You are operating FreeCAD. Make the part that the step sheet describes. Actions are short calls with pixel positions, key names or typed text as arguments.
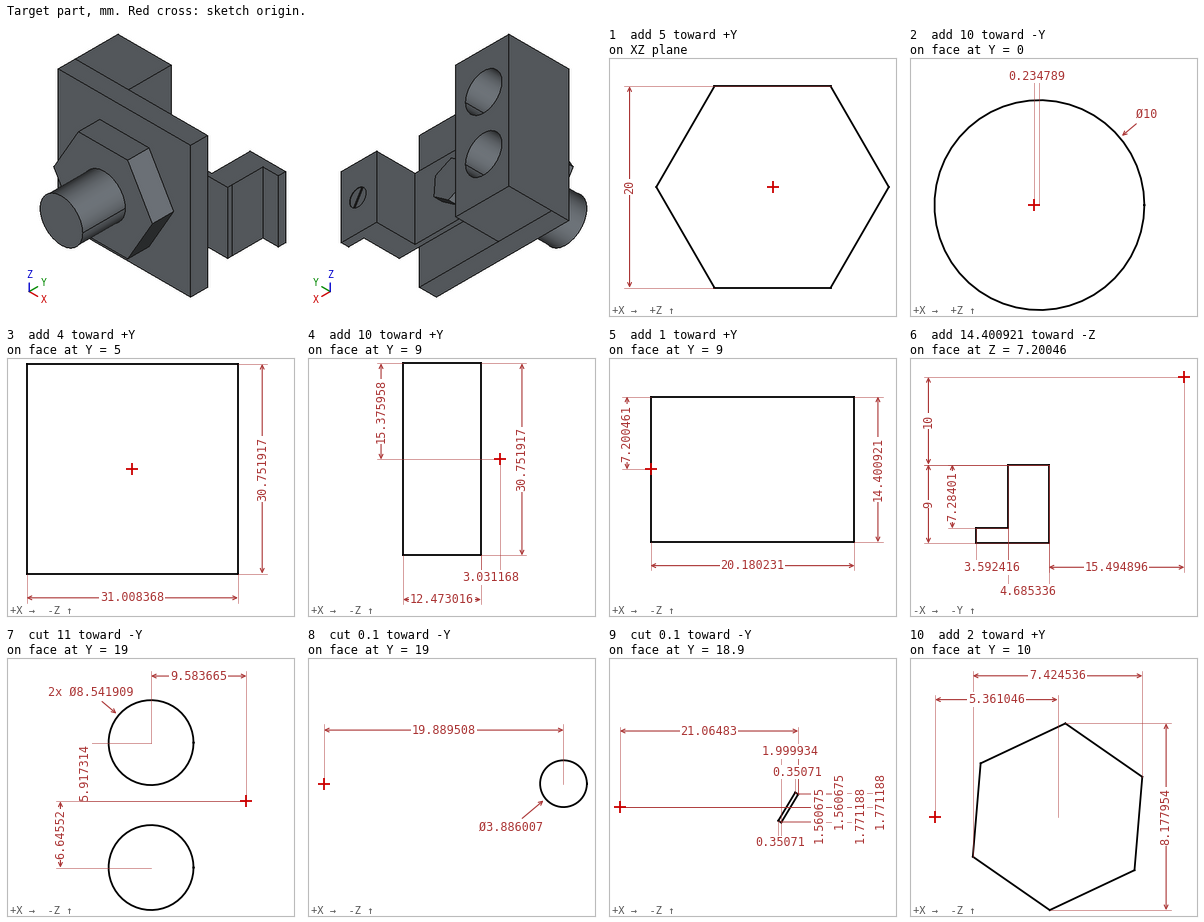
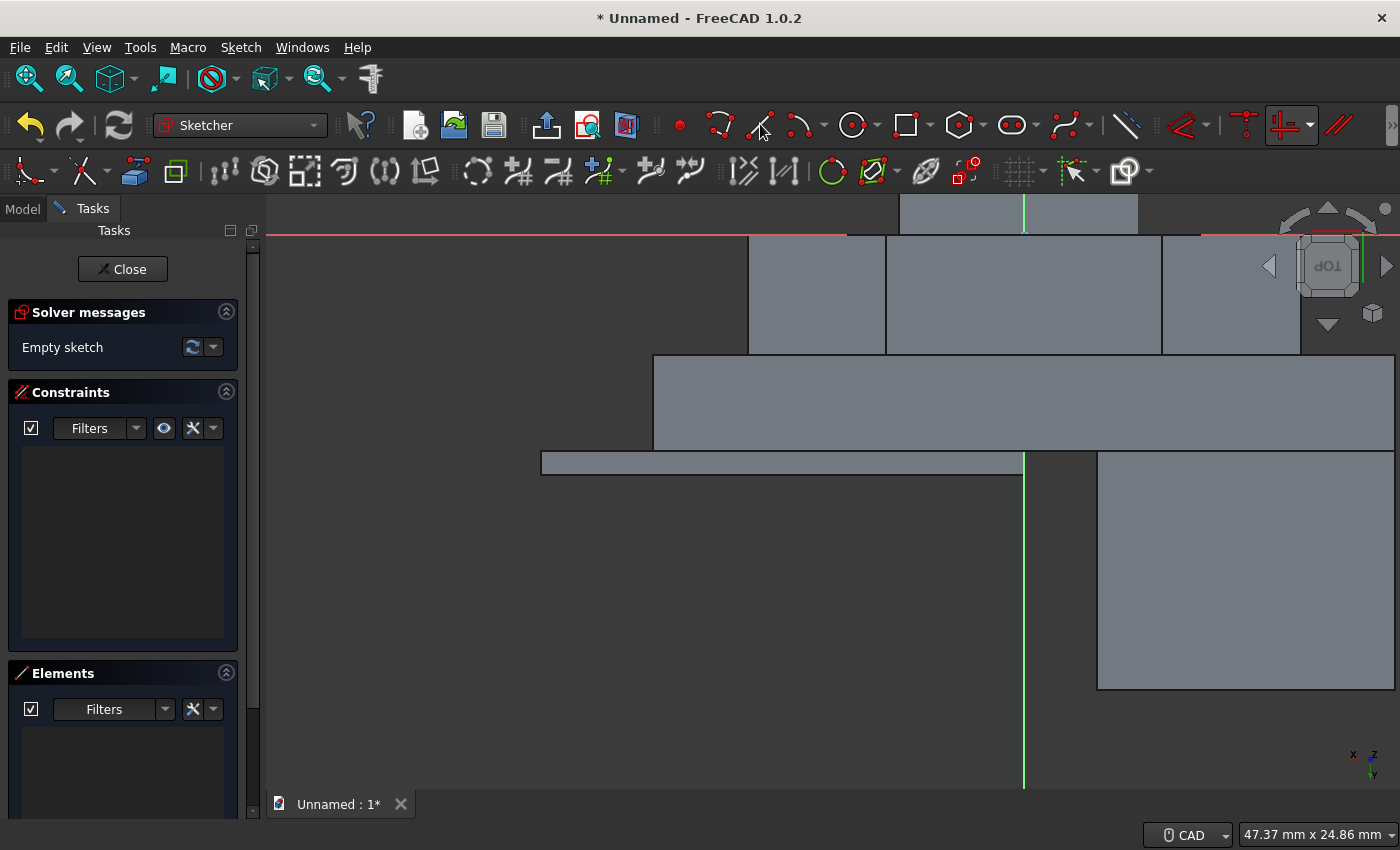
click(628, 126)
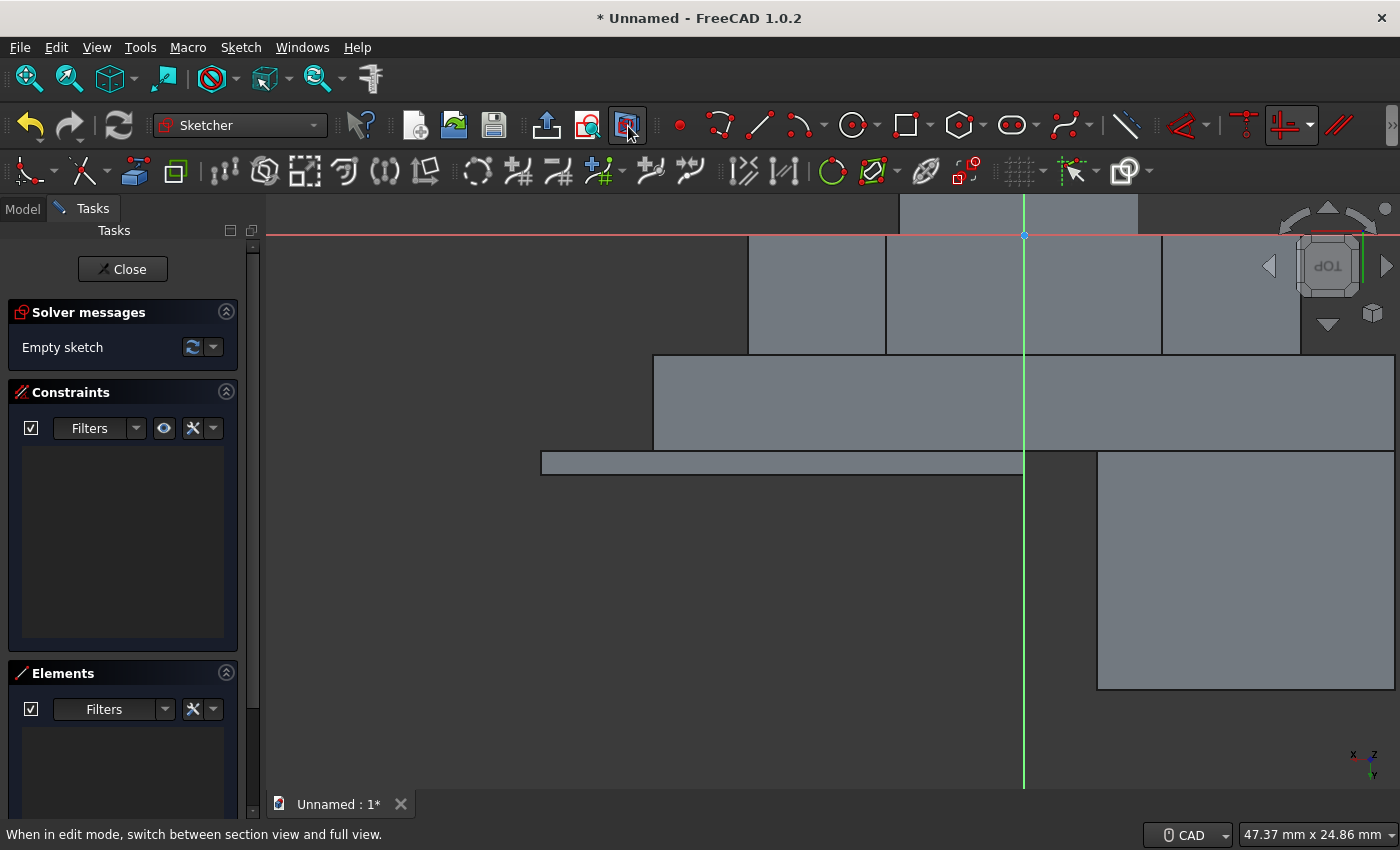
scroll(298, 693, up, 3)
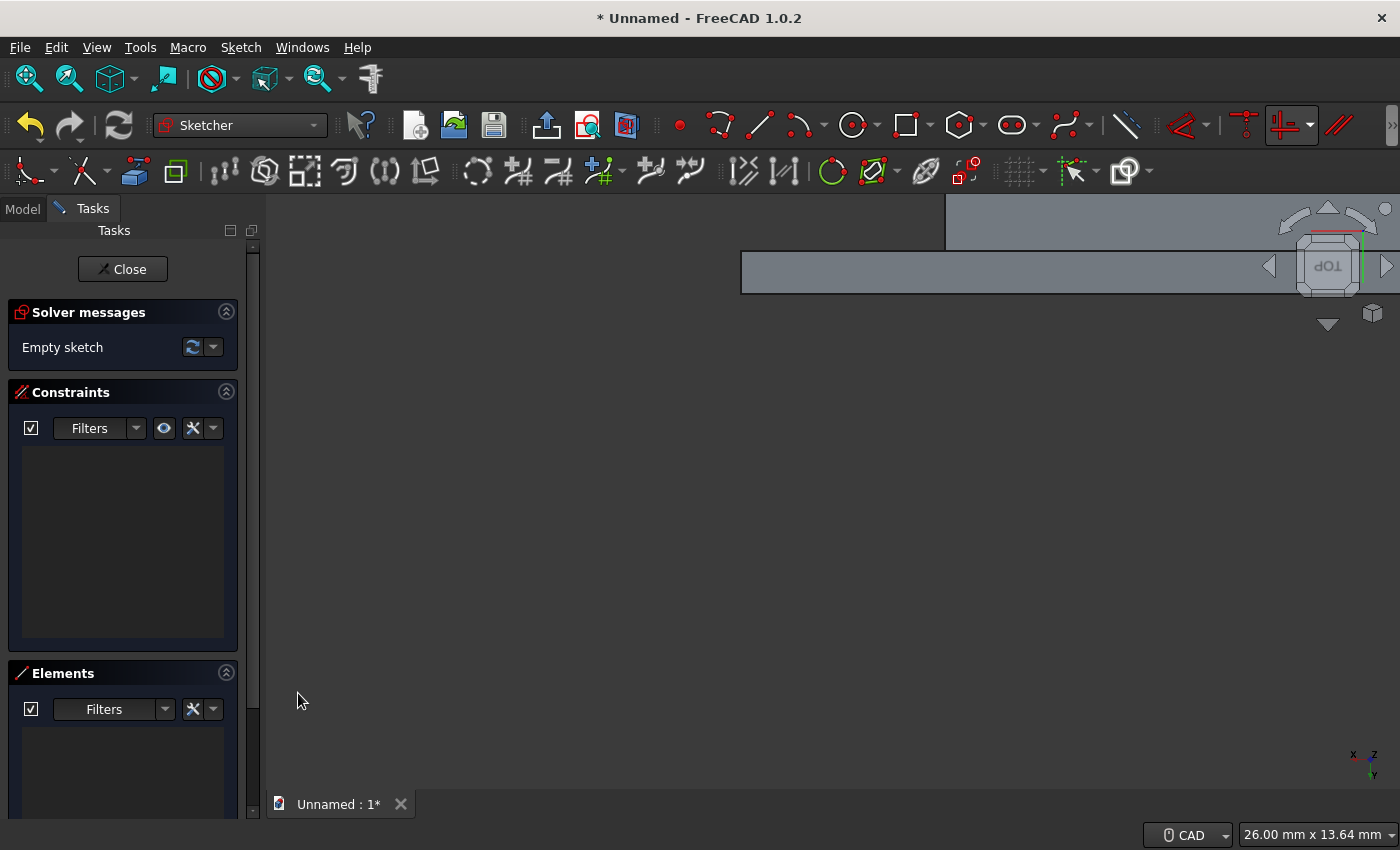
click(720, 126)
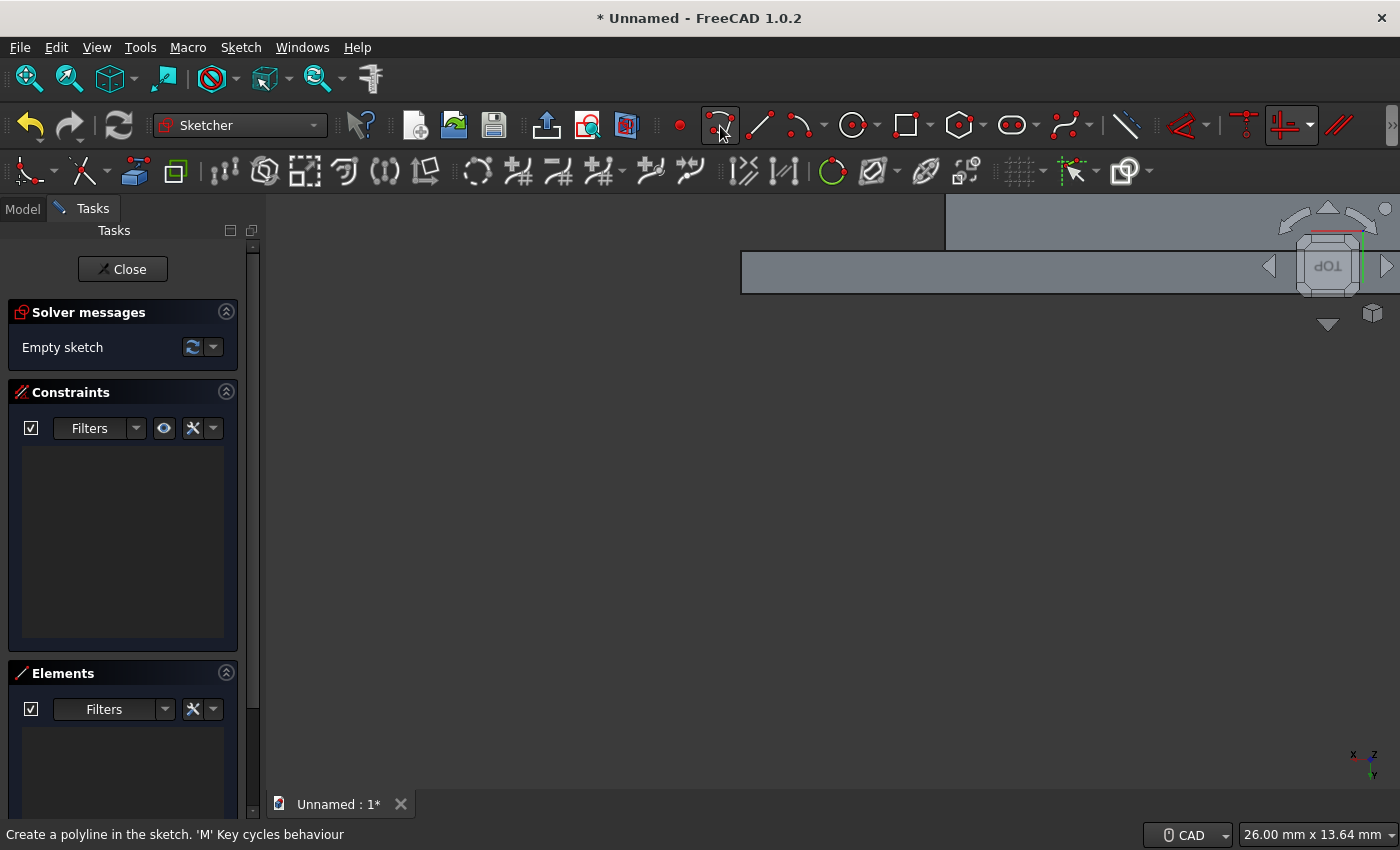
click(945, 294)
click(741, 294)
click(741, 612)
click(584, 612)
click(584, 687)
click(945, 687)
click(945, 295)
key(Escape)
key(Escape)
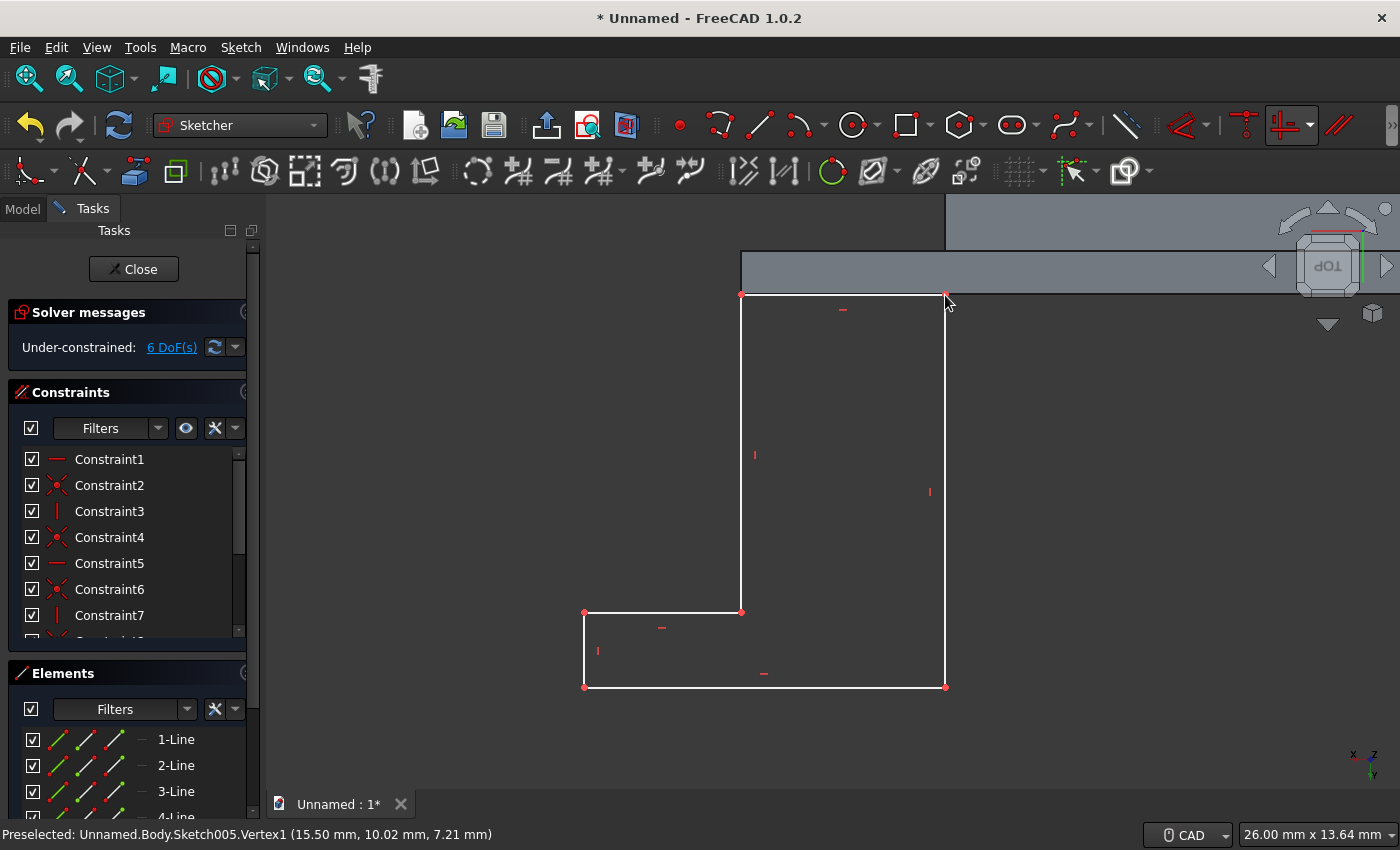
click(1182, 126)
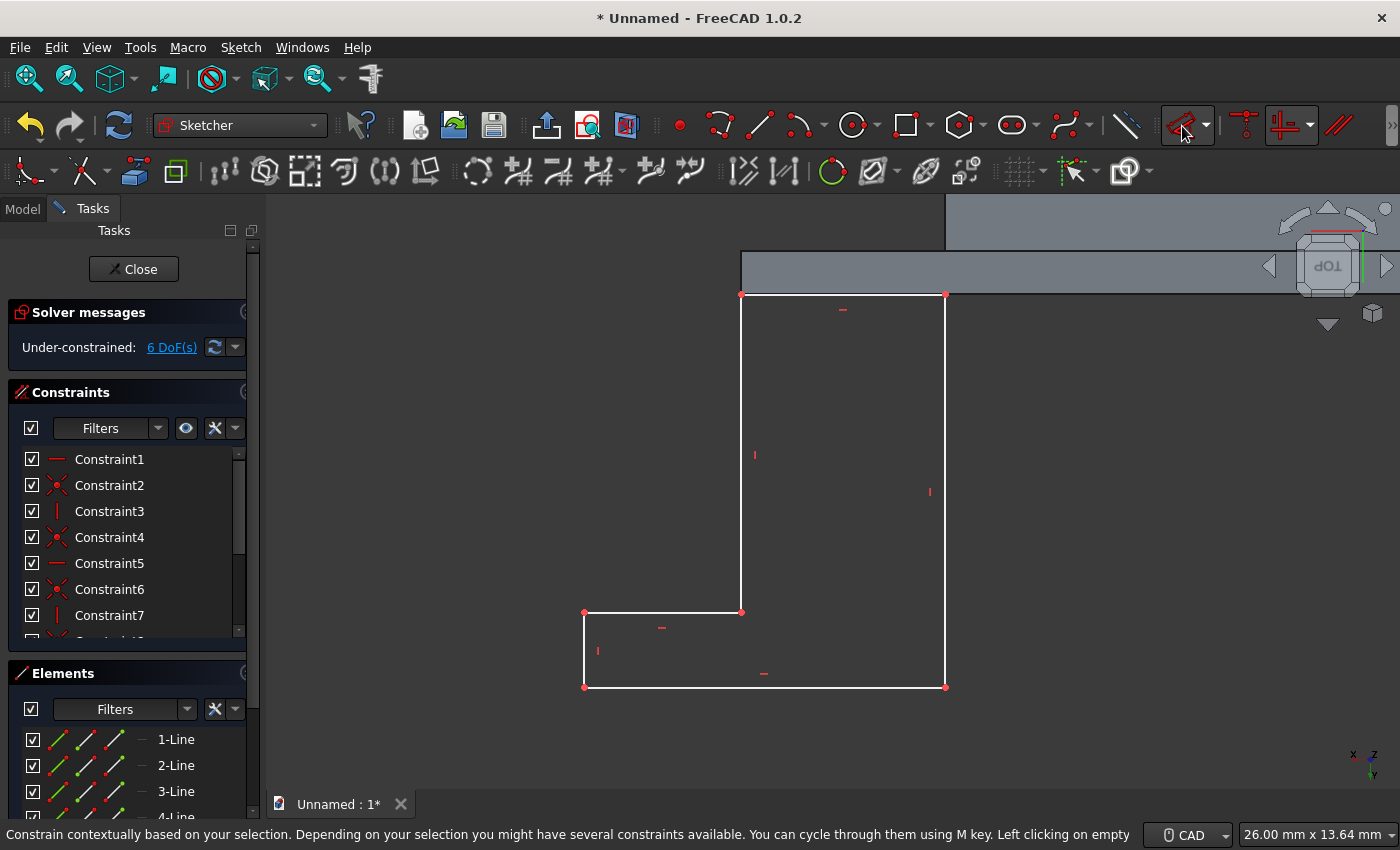
click(945, 570)
click(979, 491)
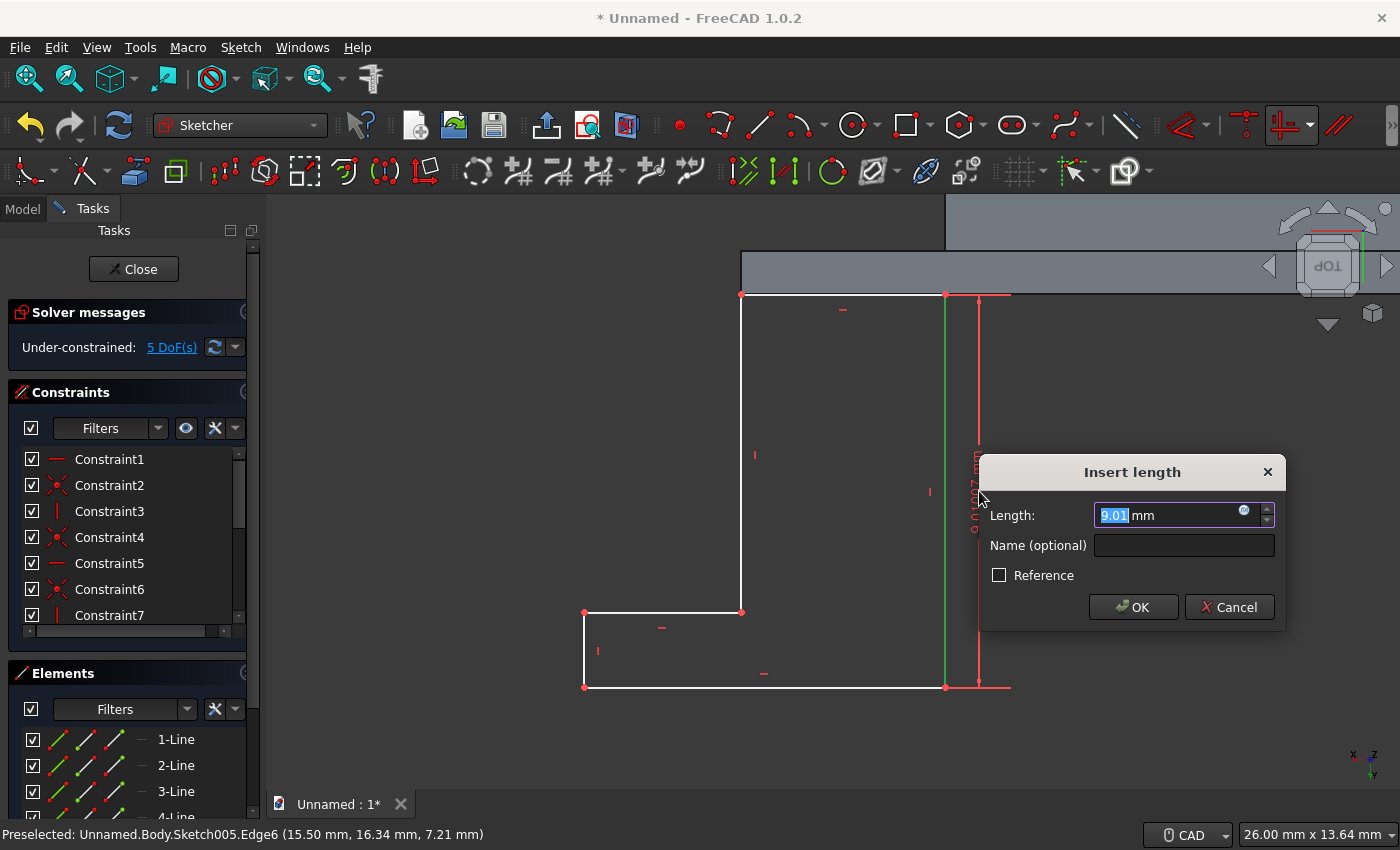
text(9)
key(Return)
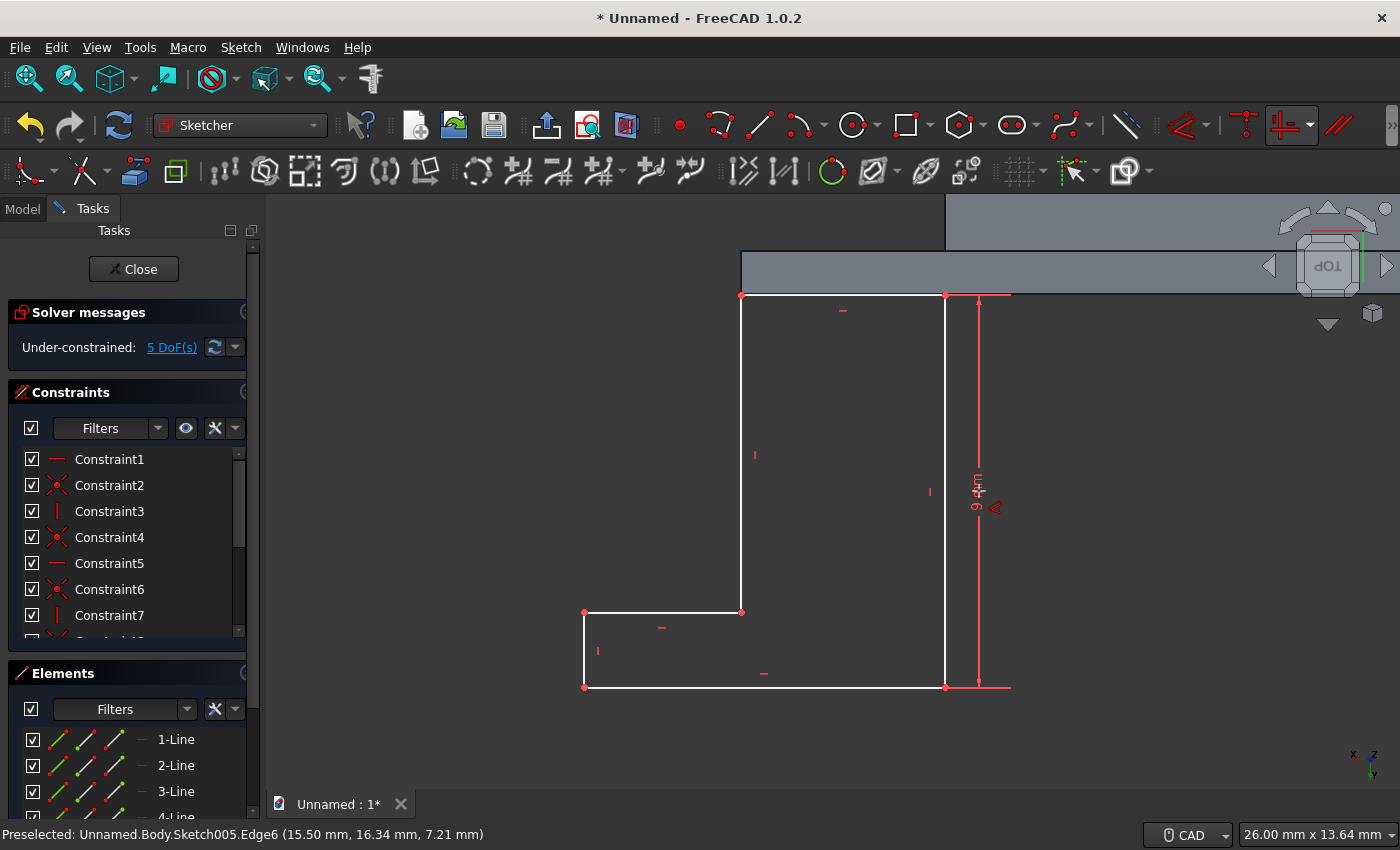
click(945, 295)
click(911, 259)